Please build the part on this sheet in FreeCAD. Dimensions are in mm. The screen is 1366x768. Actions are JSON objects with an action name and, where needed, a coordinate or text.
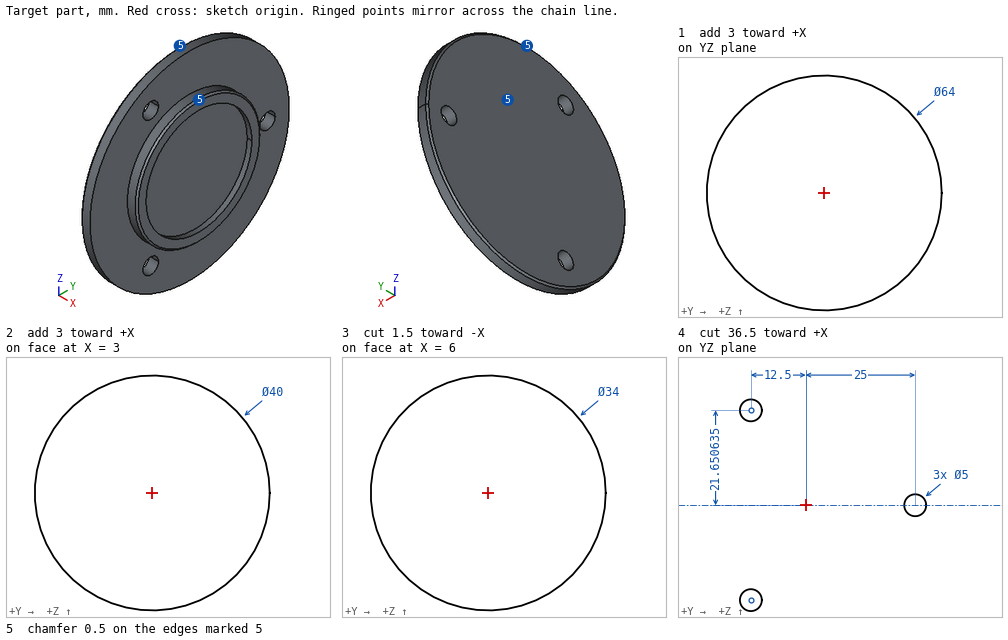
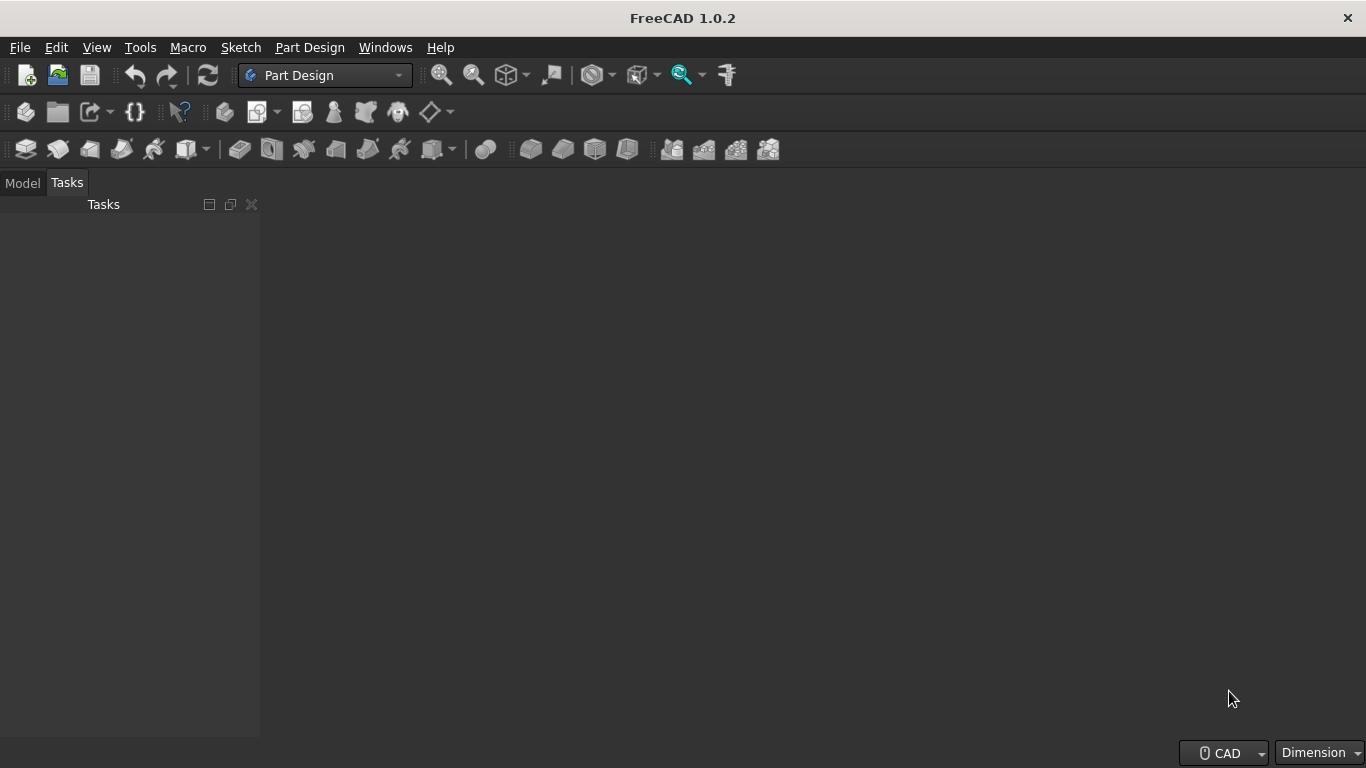
{"action": "left_click", "coordinate": [26, 76]}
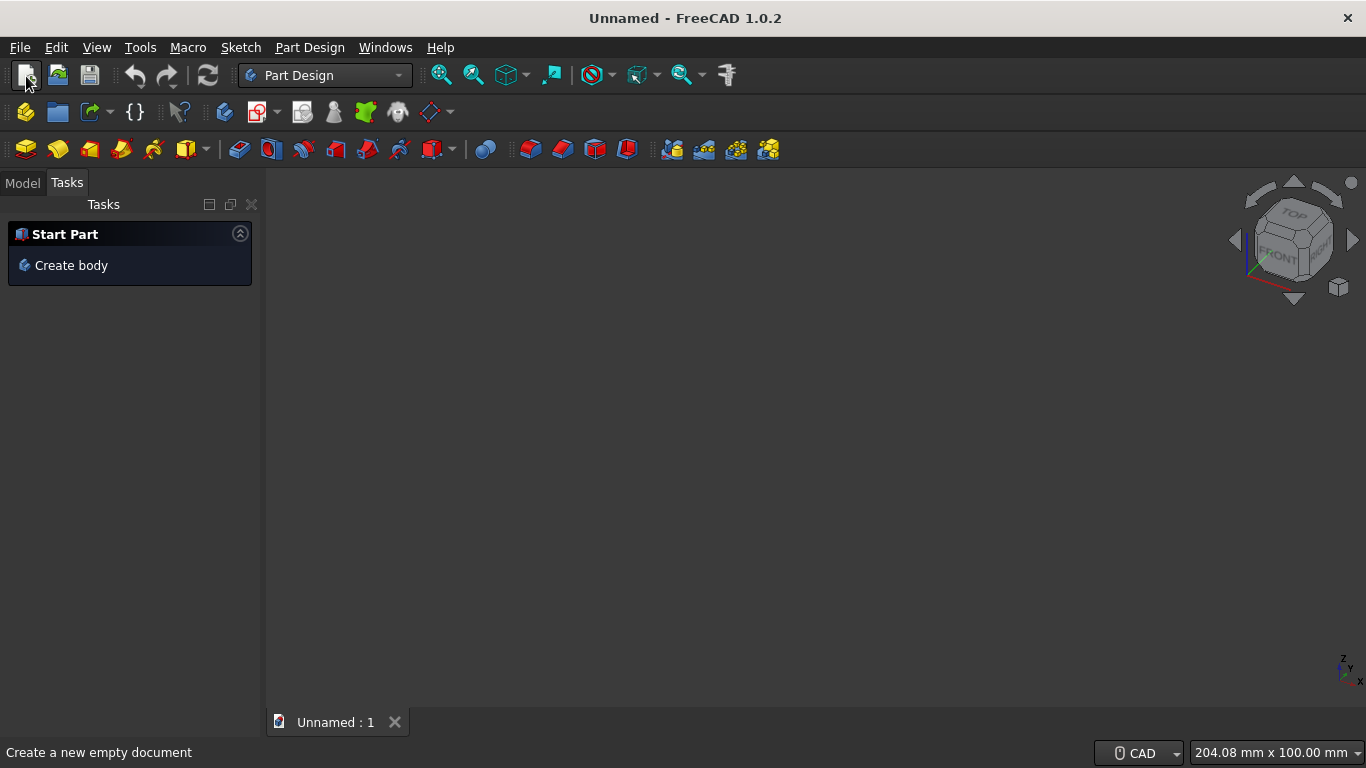
{"action": "left_click", "coordinate": [258, 112]}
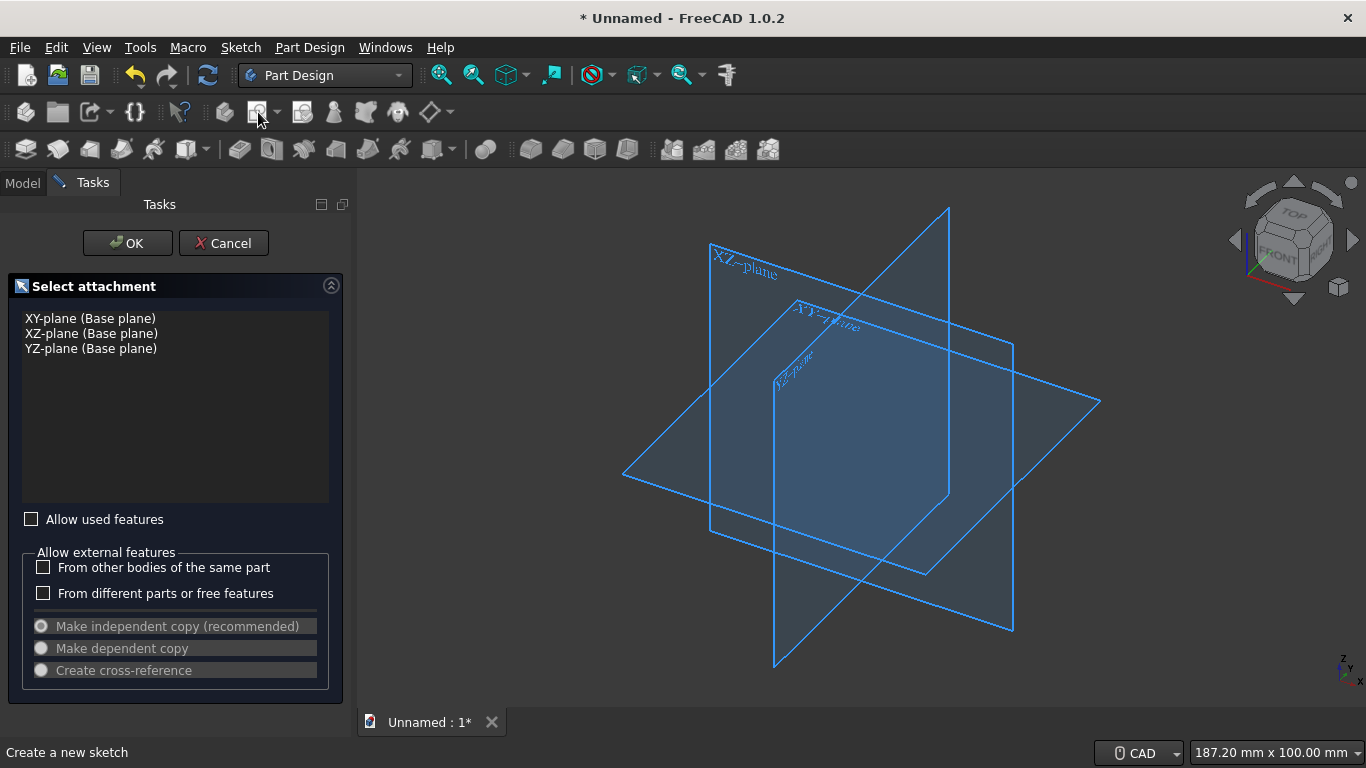
{"action": "left_click", "coordinate": [82, 348]}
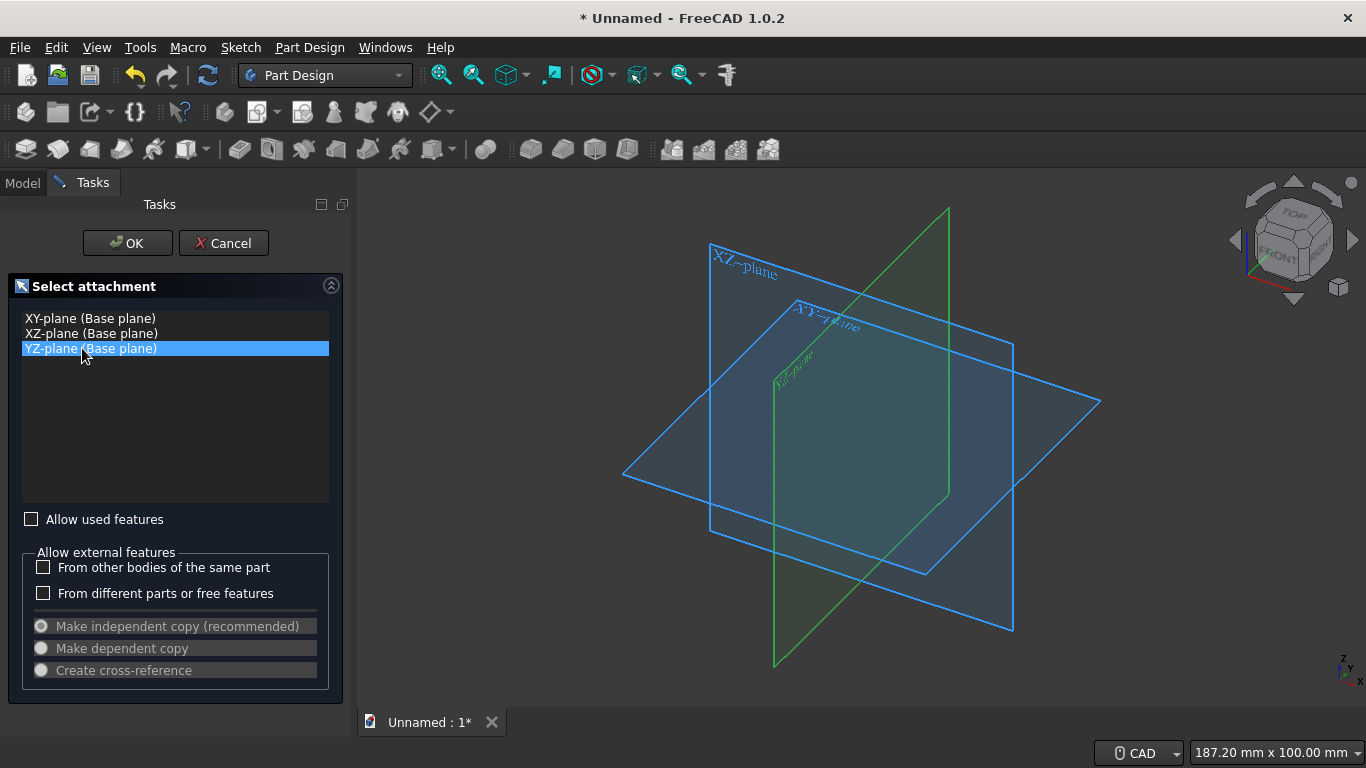
{"action": "left_click", "coordinate": [128, 243]}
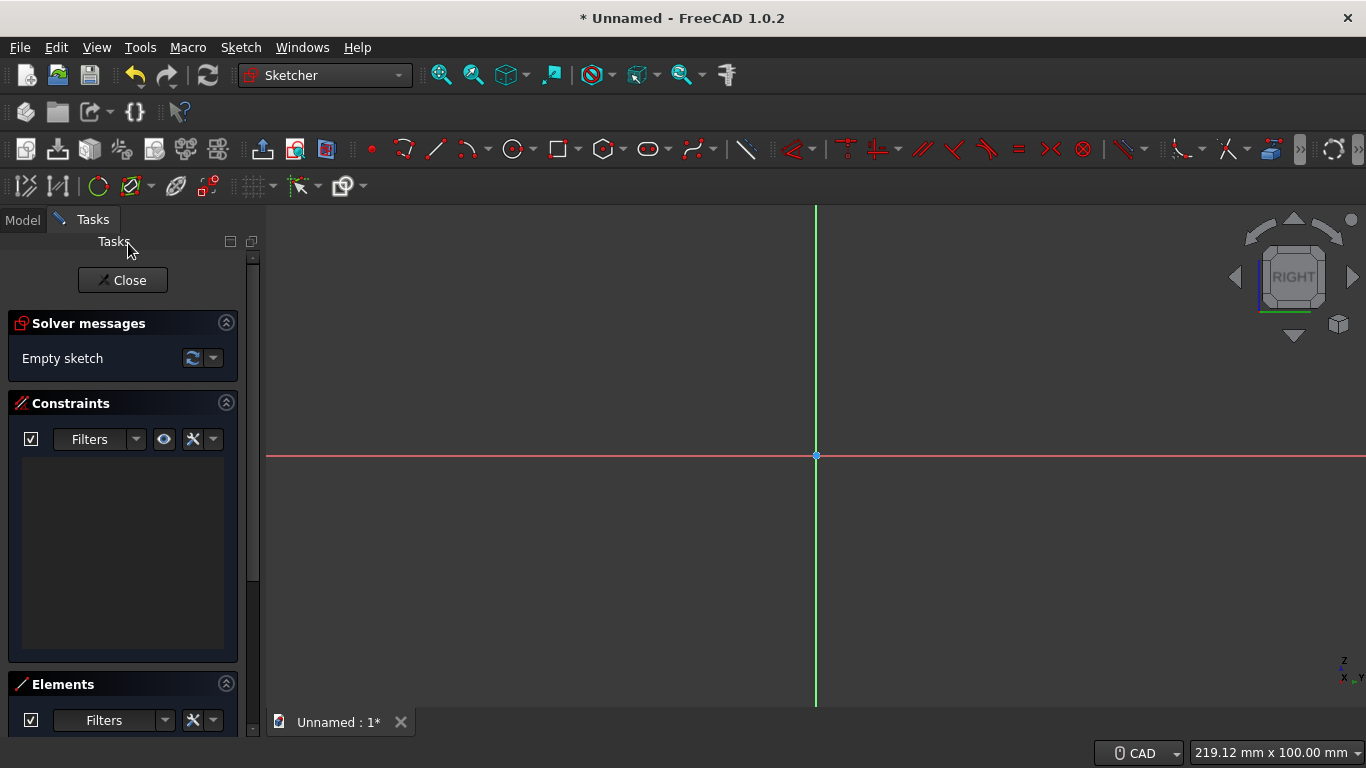
{"action": "key", "text": "g c"}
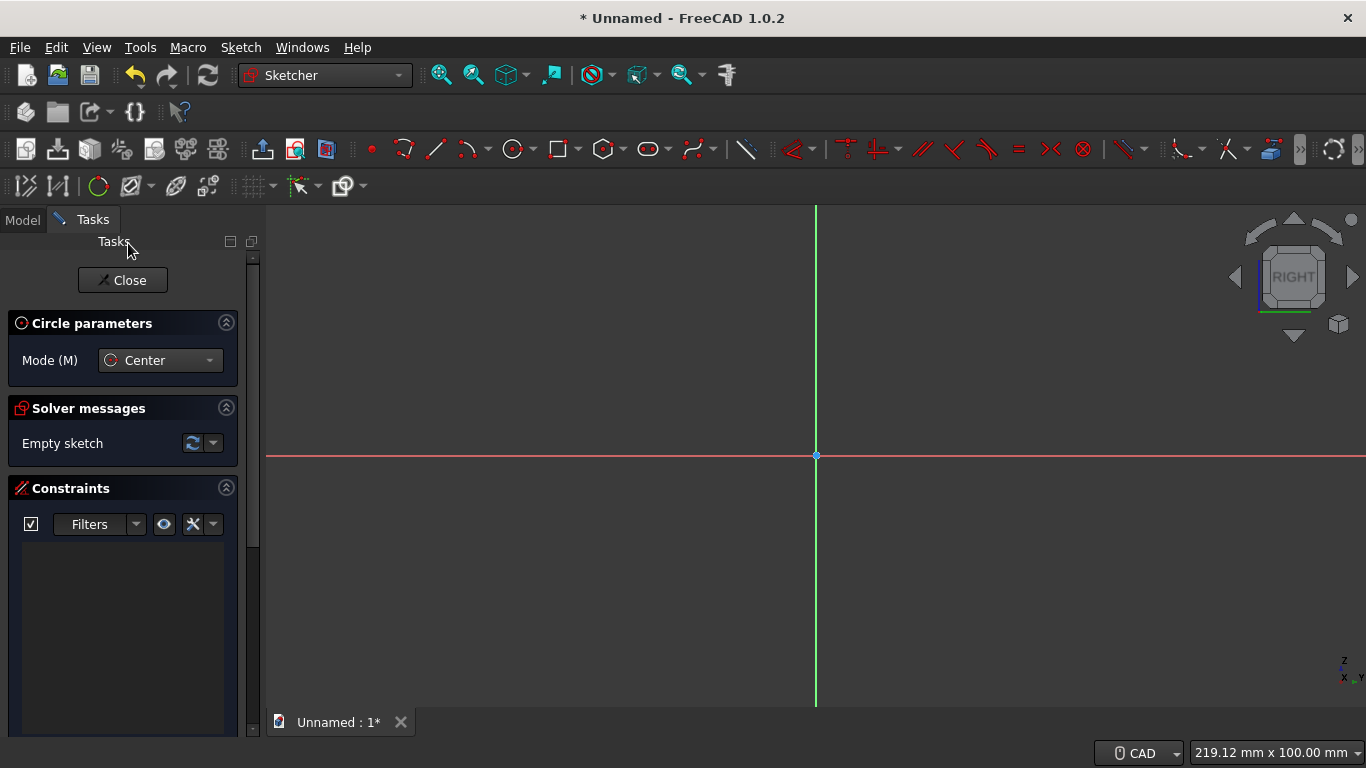
{"action": "left_click", "coordinate": [816, 456]}
{"action": "left_click", "coordinate": [930, 342]}
{"action": "key", "text": "Escape"}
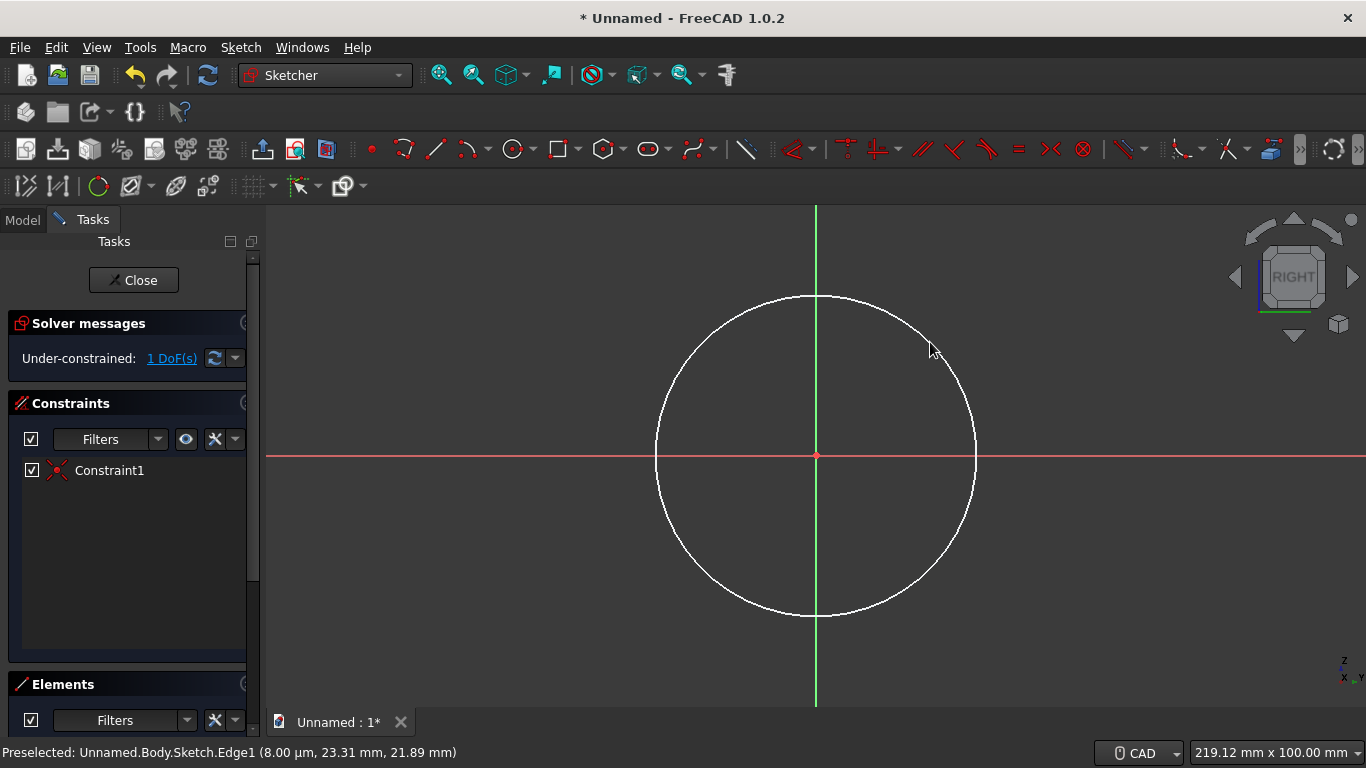
{"action": "left_click", "coordinate": [929, 342]}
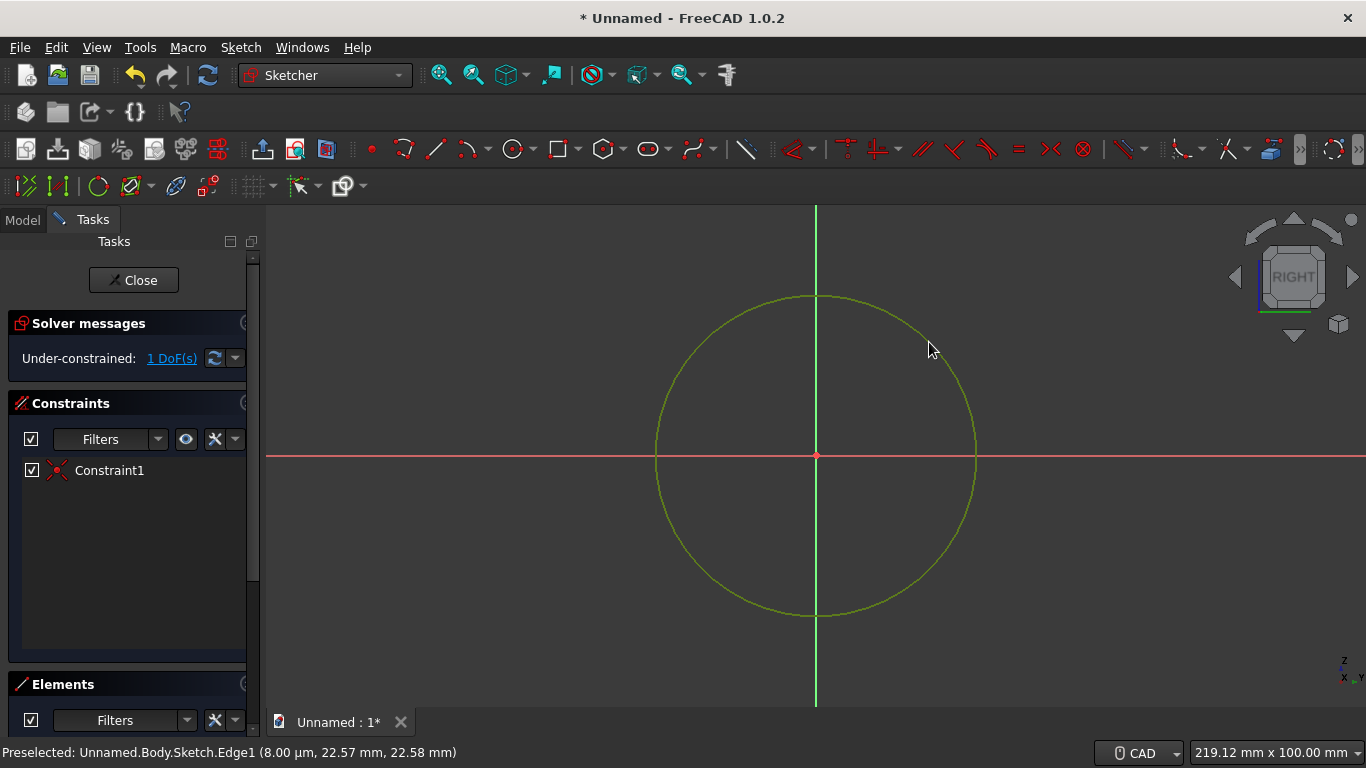
{"action": "left_click", "coordinate": [814, 150]}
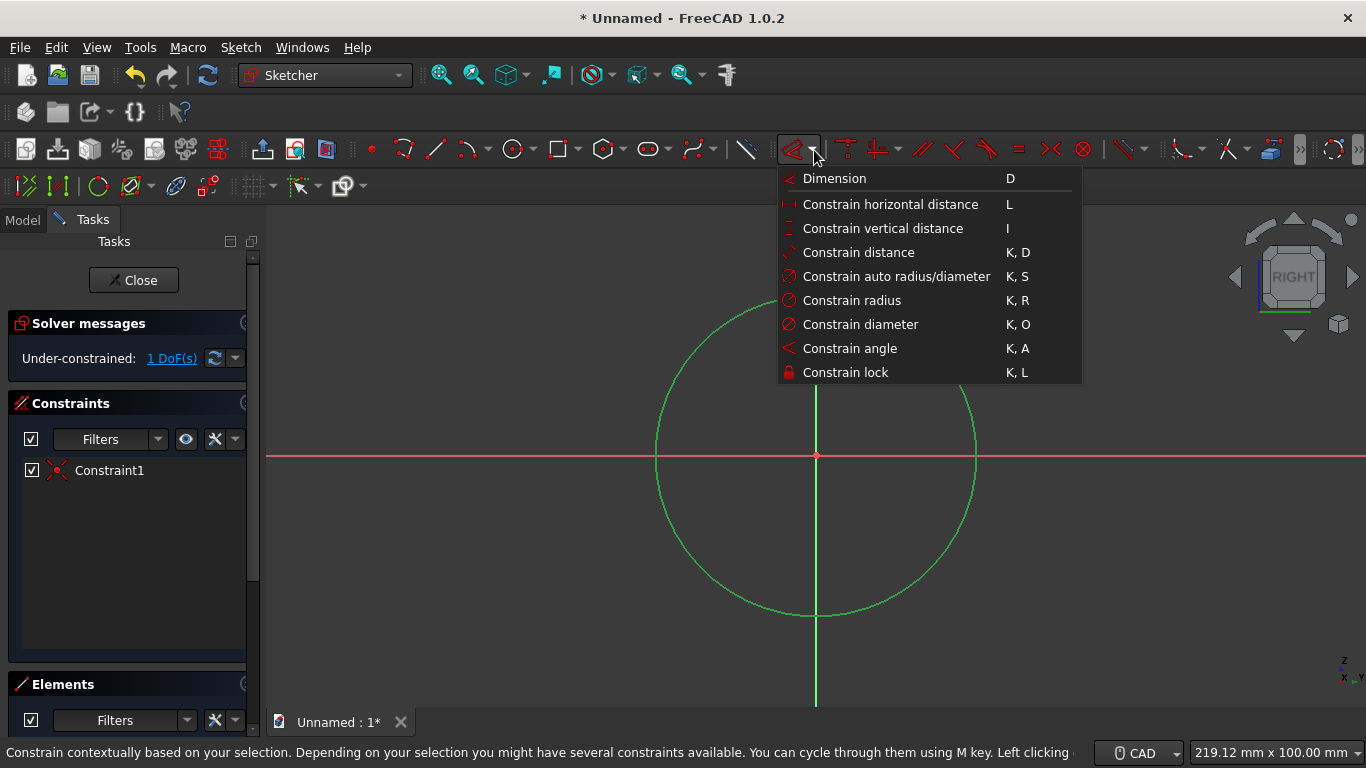
{"action": "left_click", "coordinate": [930, 324]}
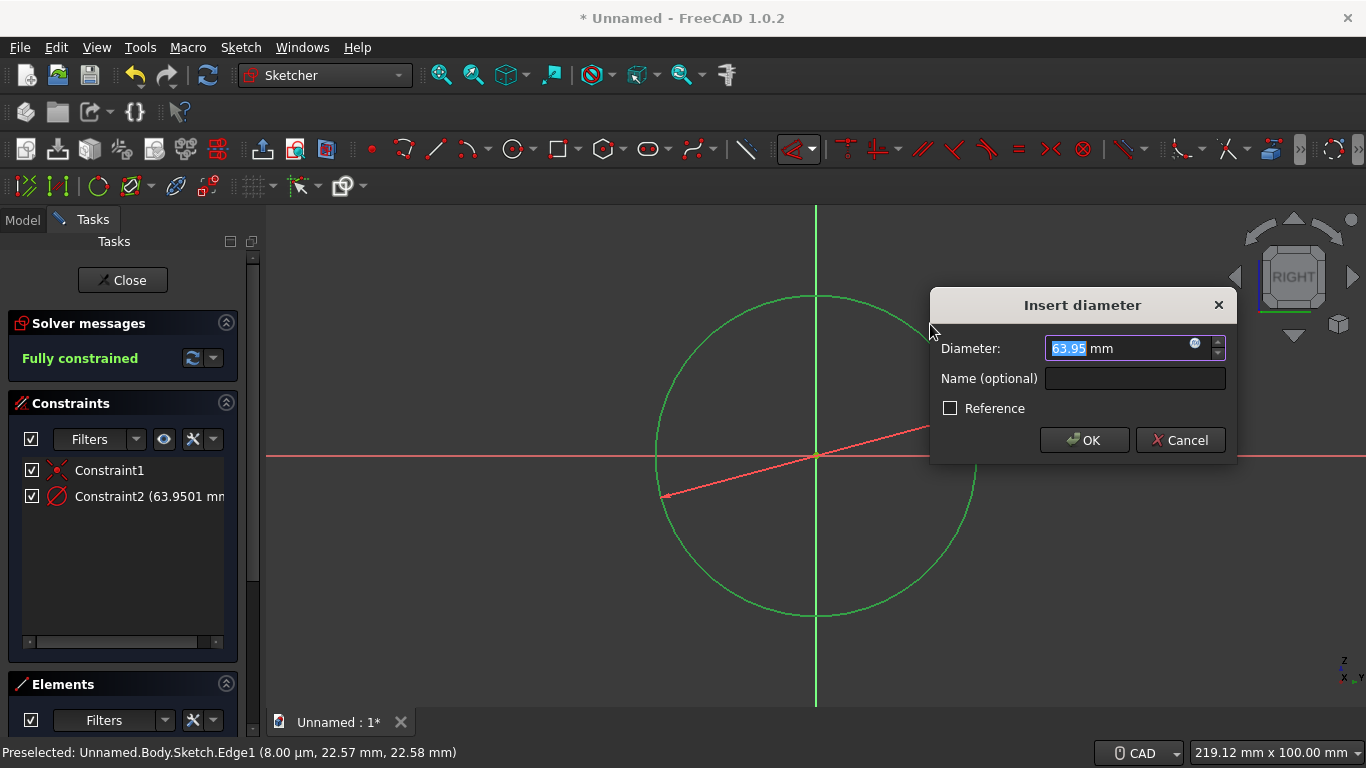
{"action": "type", "text": "64"}
{"action": "key", "text": "Return"}